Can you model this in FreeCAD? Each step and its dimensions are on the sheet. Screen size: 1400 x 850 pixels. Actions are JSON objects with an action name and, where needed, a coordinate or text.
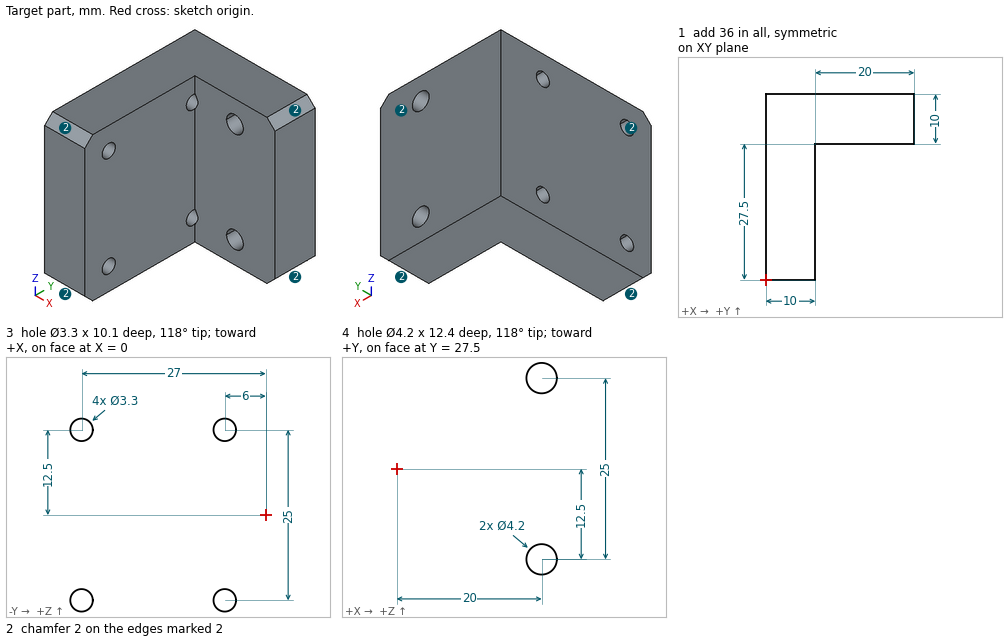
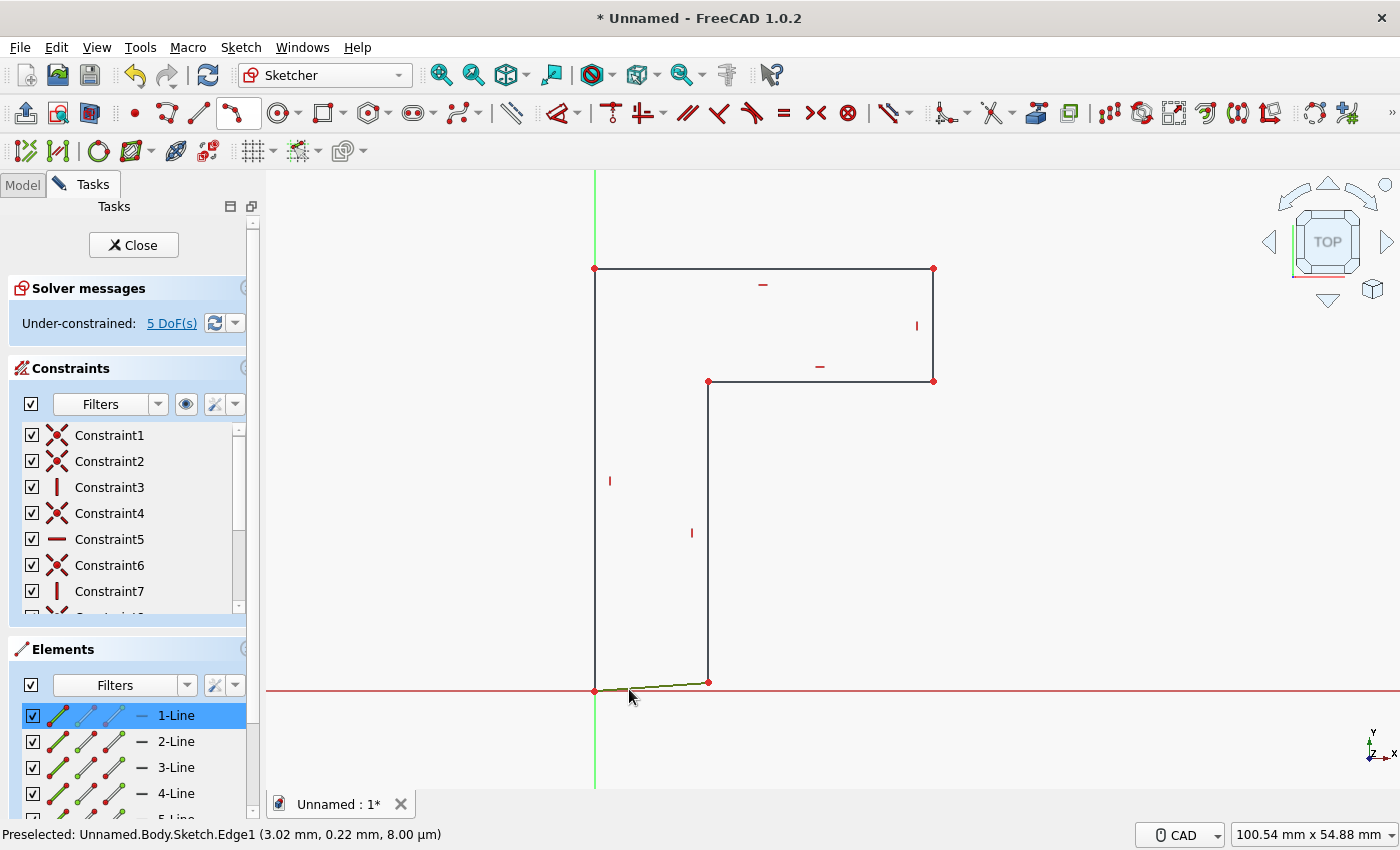
{"action": "key", "text": "h"}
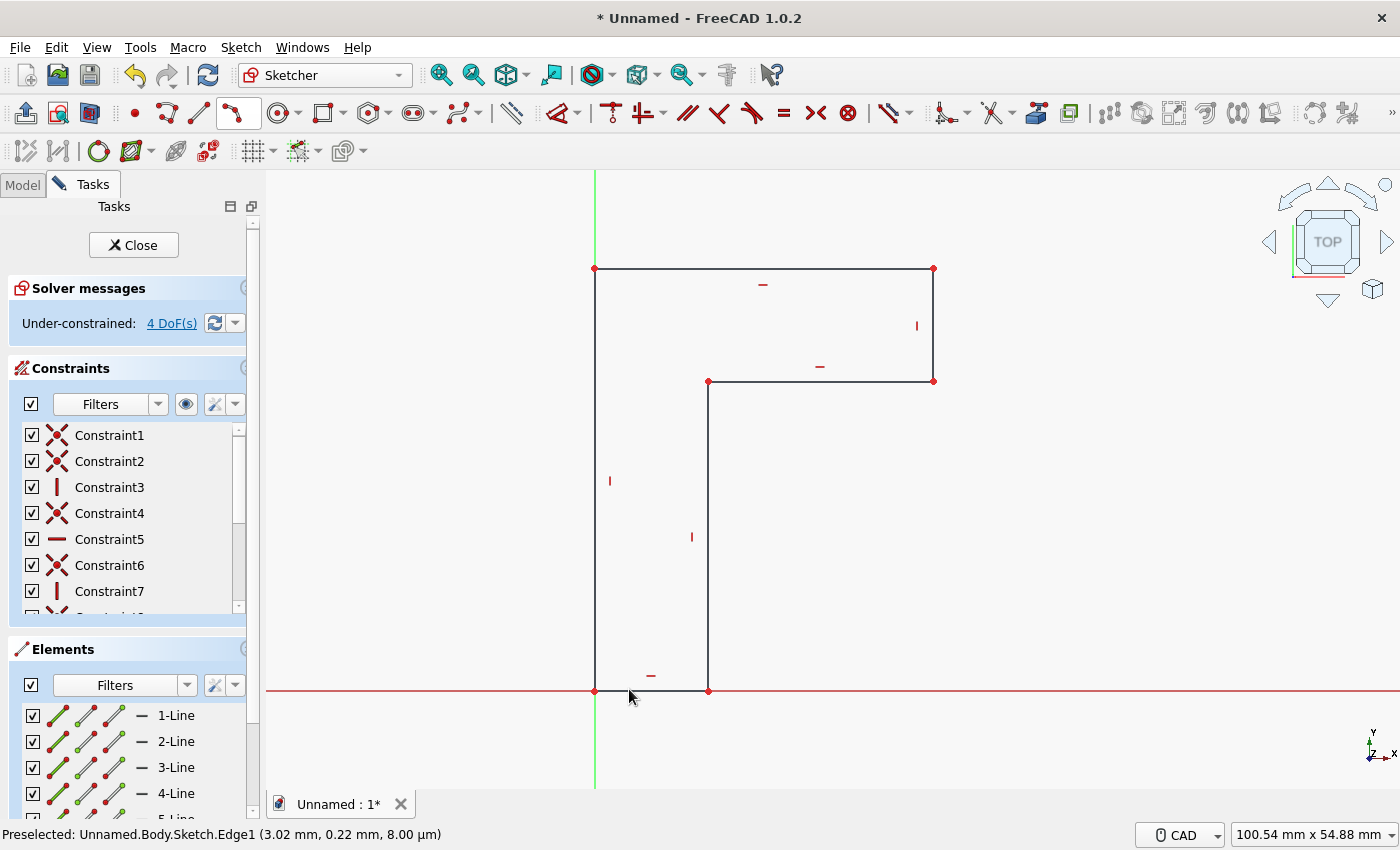
{"action": "key", "text": "d"}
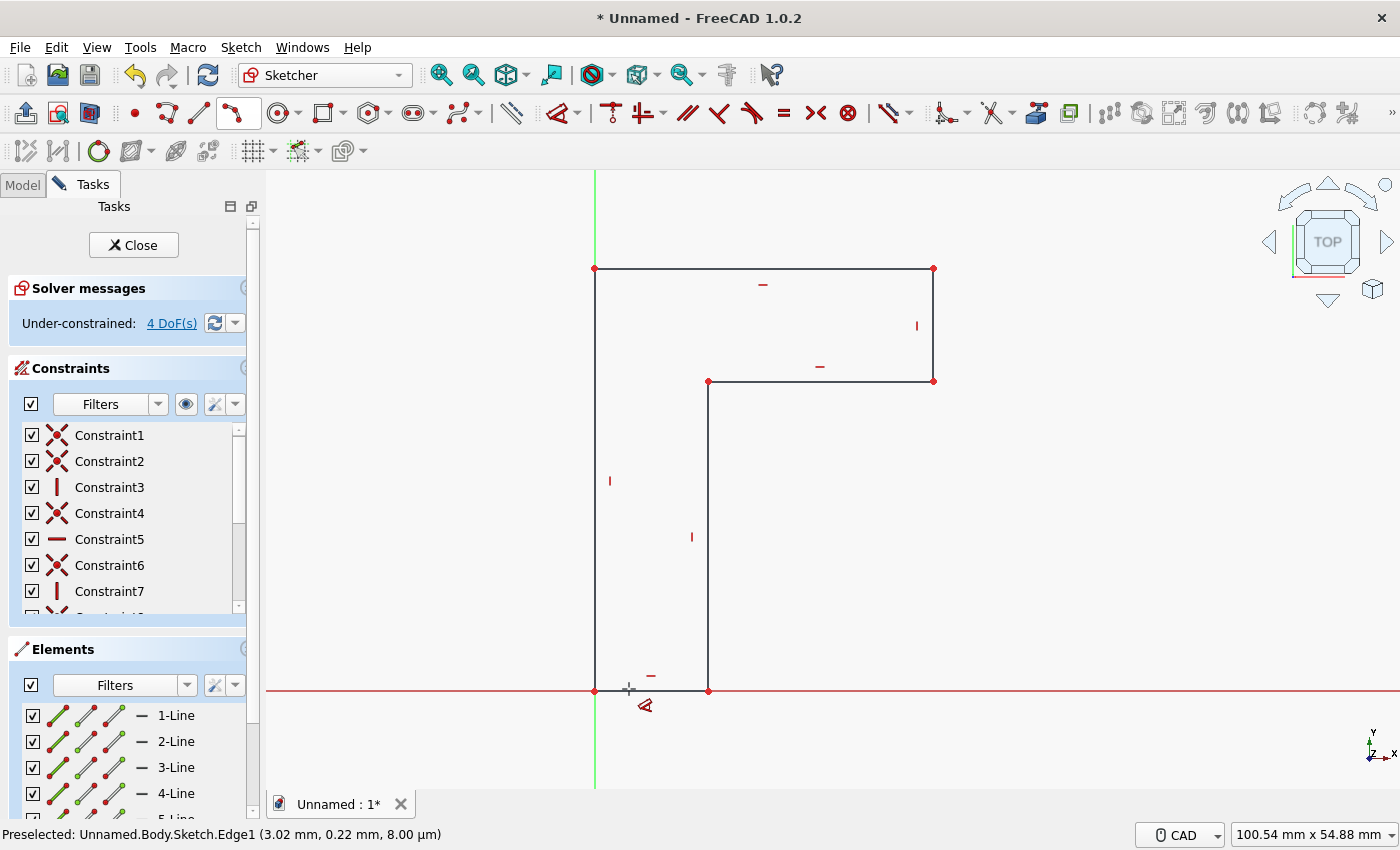
{"action": "left_click", "coordinate": [629, 691]}
{"action": "left_click", "coordinate": [651, 725]}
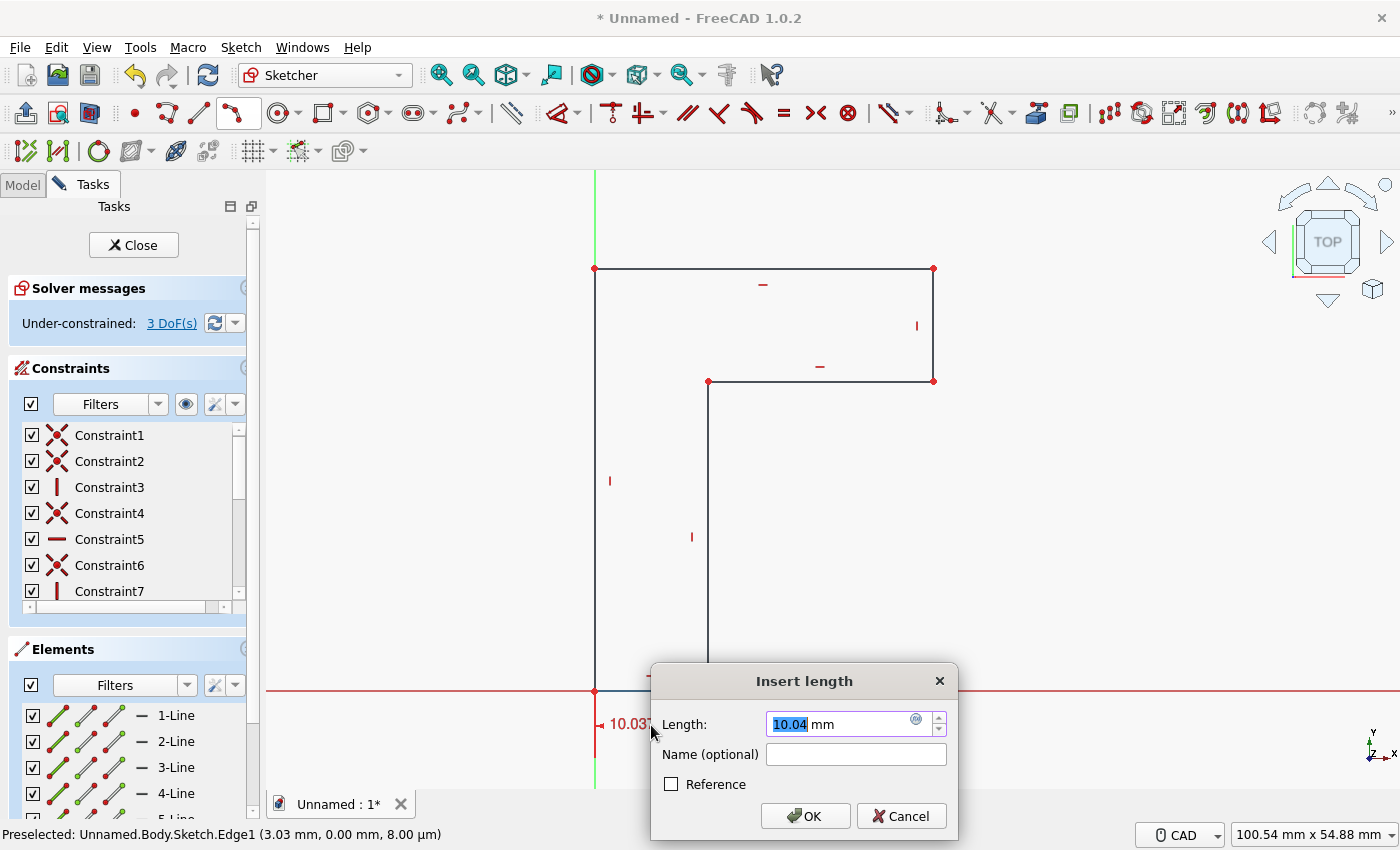
{"action": "type", "text": "10"}
{"action": "key", "text": "Return"}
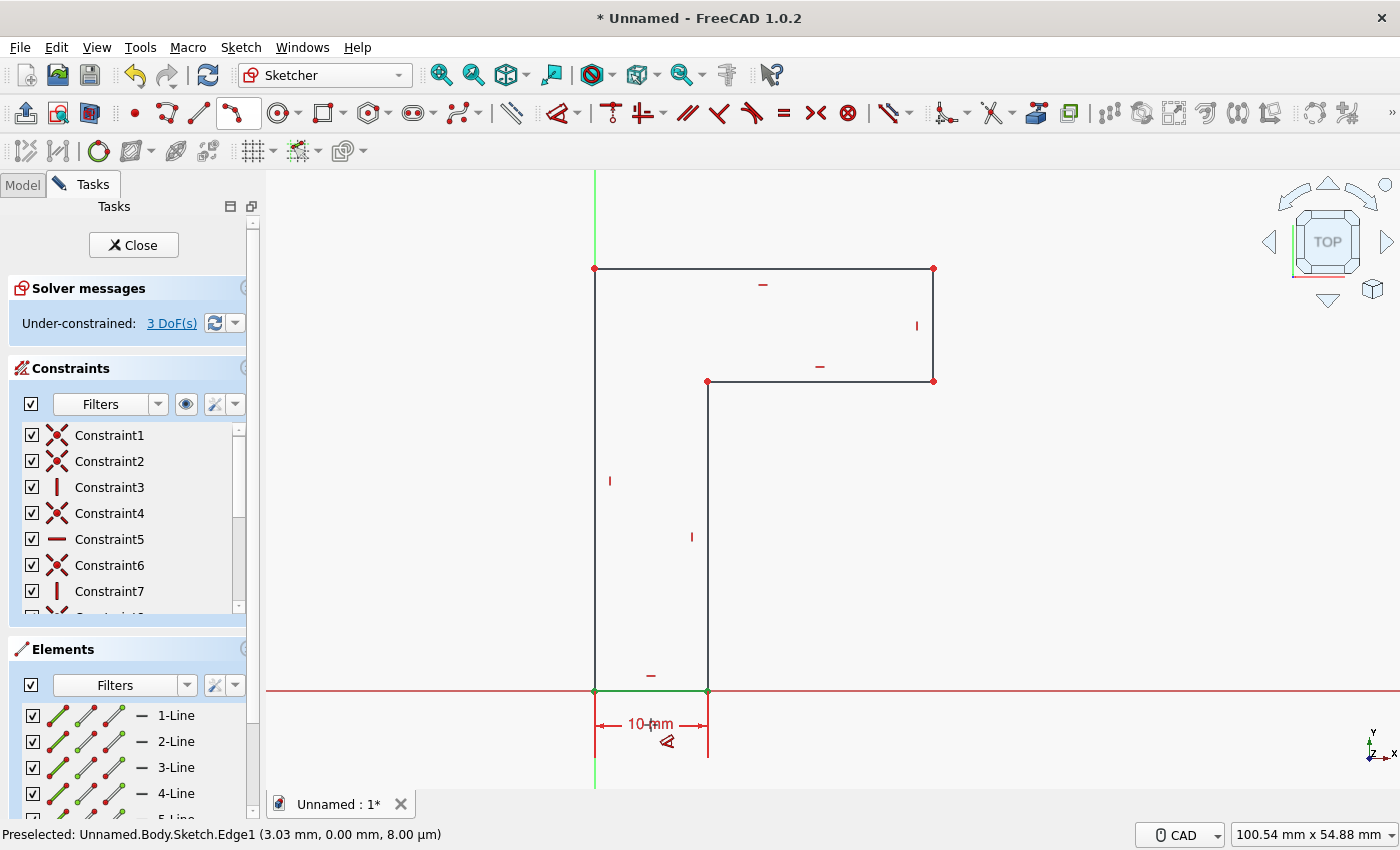
{"action": "left_click", "coordinate": [775, 382]}
{"action": "left_click", "coordinate": [820, 348]}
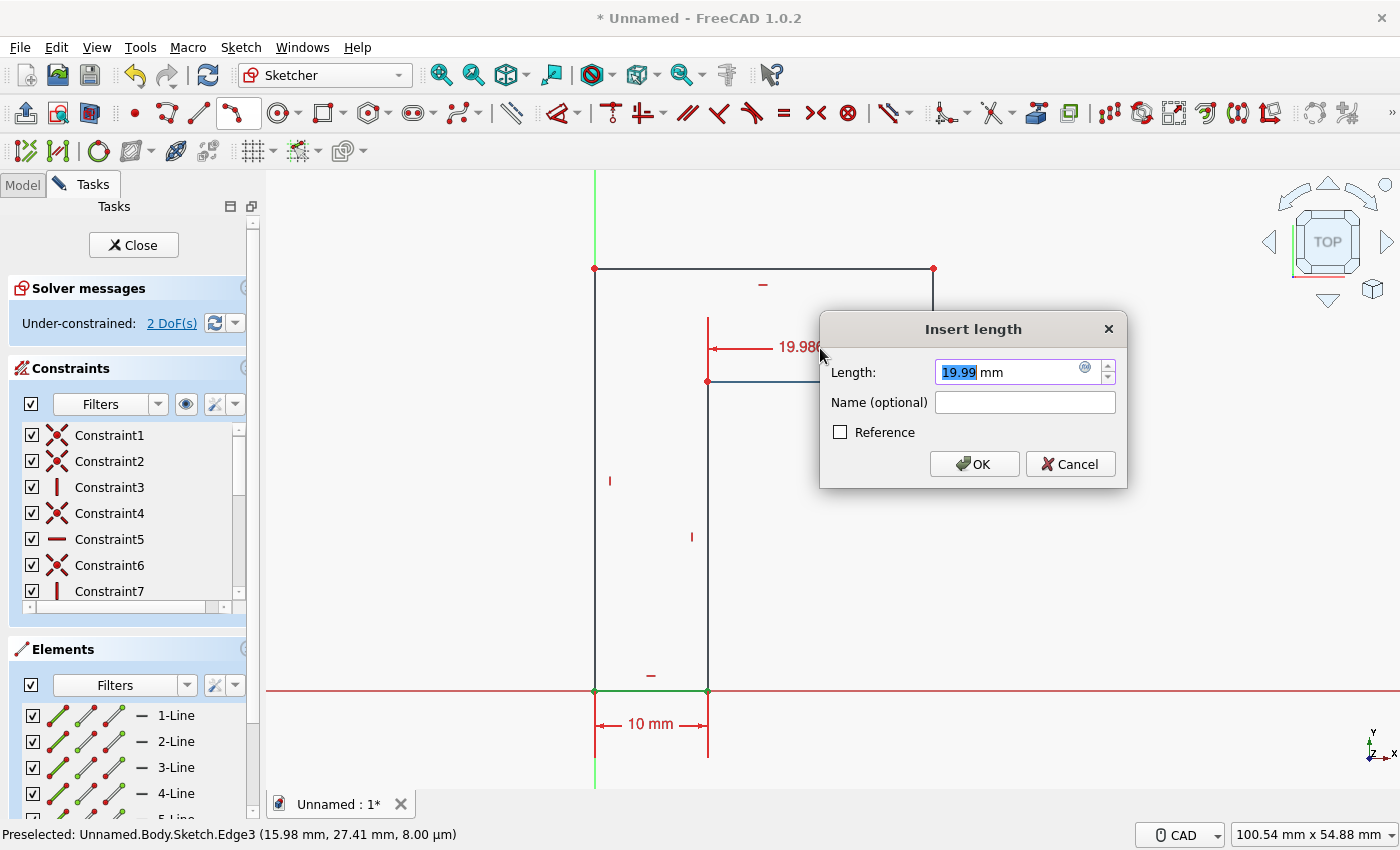
{"action": "type", "text": "20"}
{"action": "key", "text": "Return"}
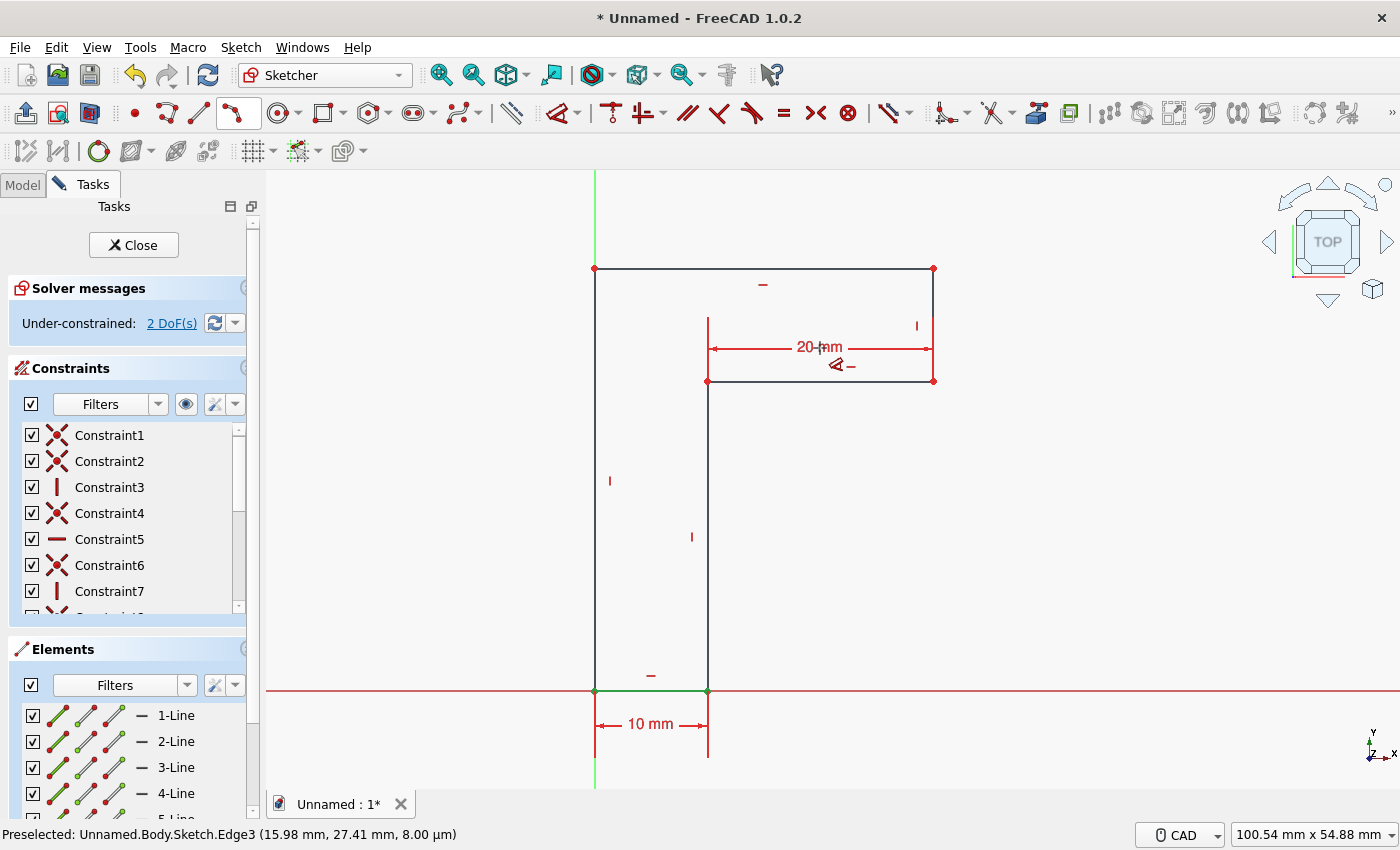
{"action": "left_click", "coordinate": [933, 348]}
{"action": "left_click", "coordinate": [967, 325]}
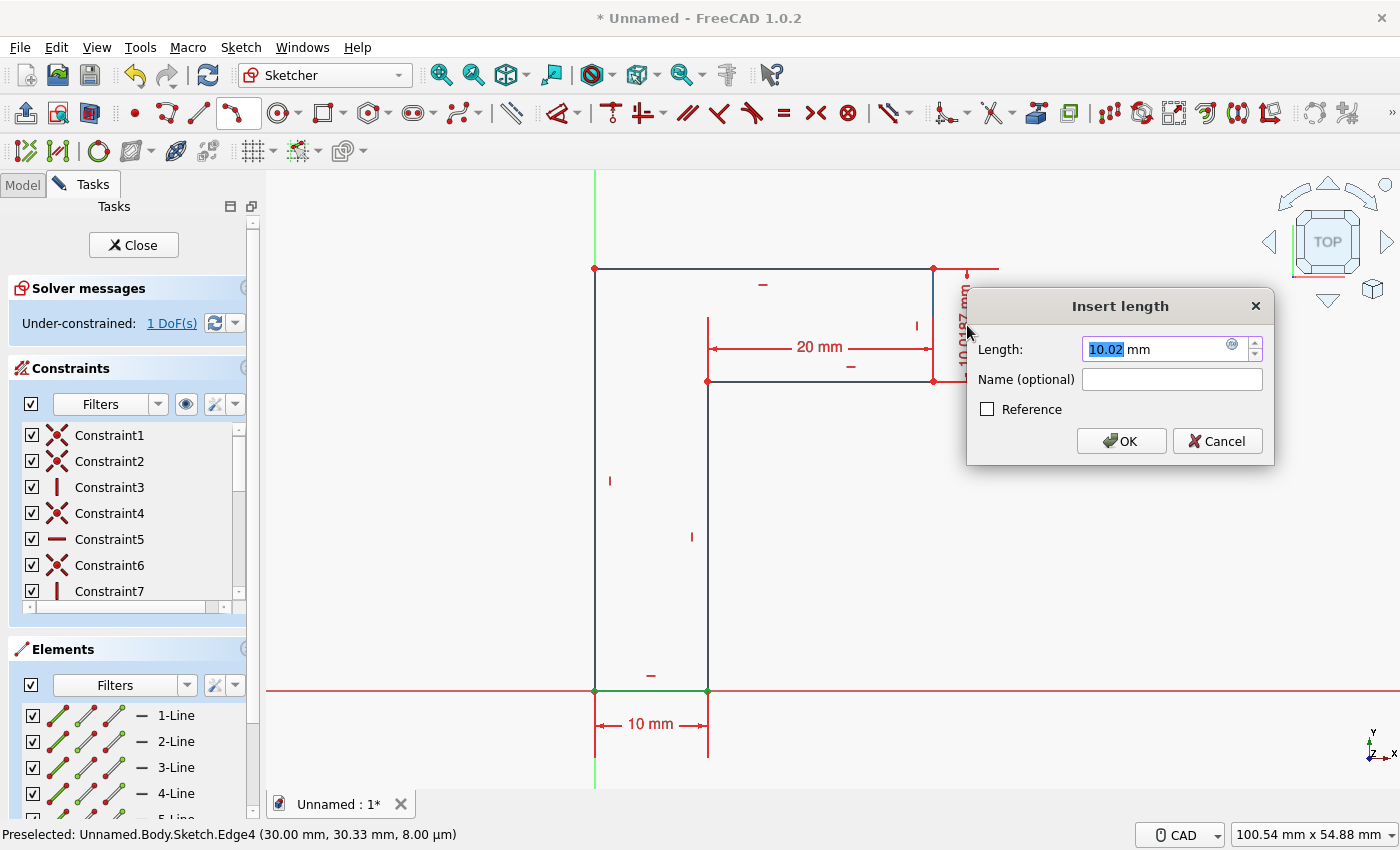
{"action": "type", "text": "10"}
{"action": "key", "text": "Return"}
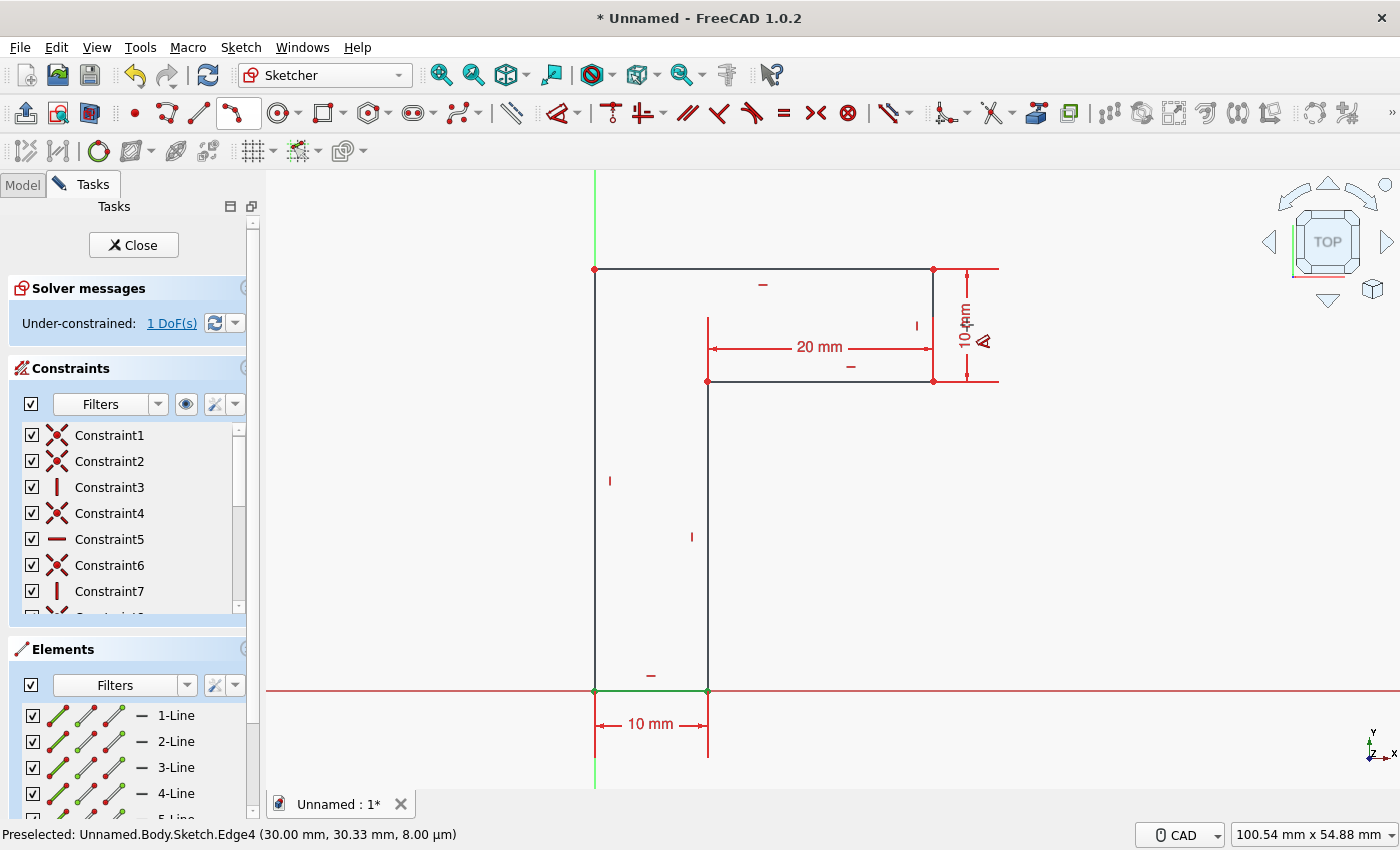
{"action": "left_click", "coordinate": [708, 598]}
{"action": "left_click", "coordinate": [674, 537]}